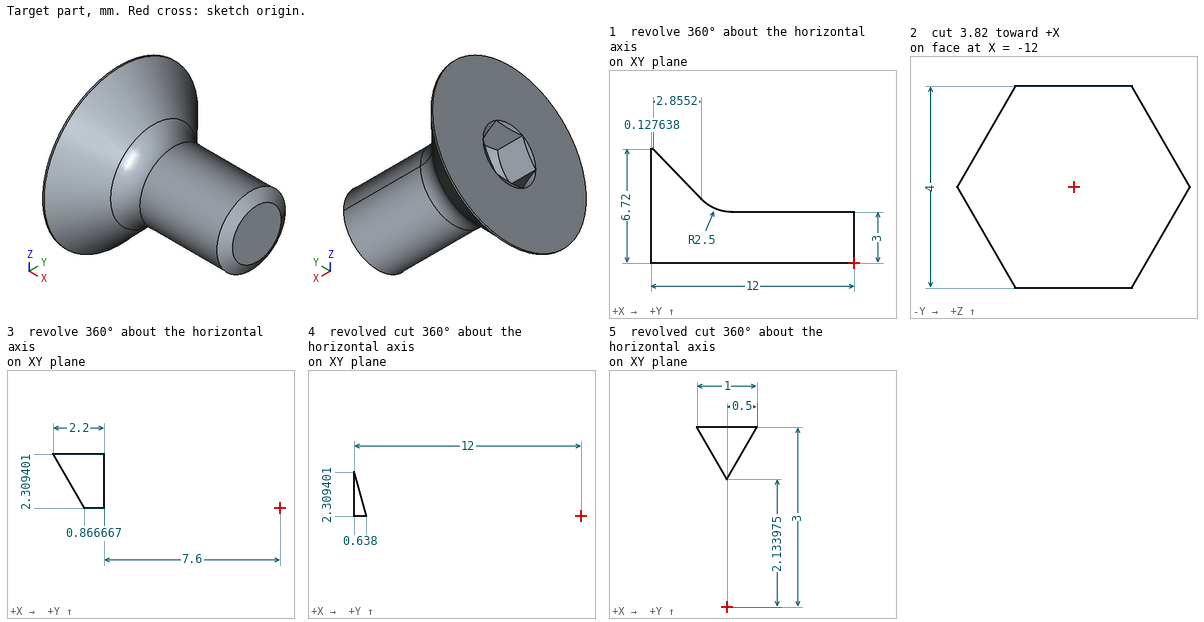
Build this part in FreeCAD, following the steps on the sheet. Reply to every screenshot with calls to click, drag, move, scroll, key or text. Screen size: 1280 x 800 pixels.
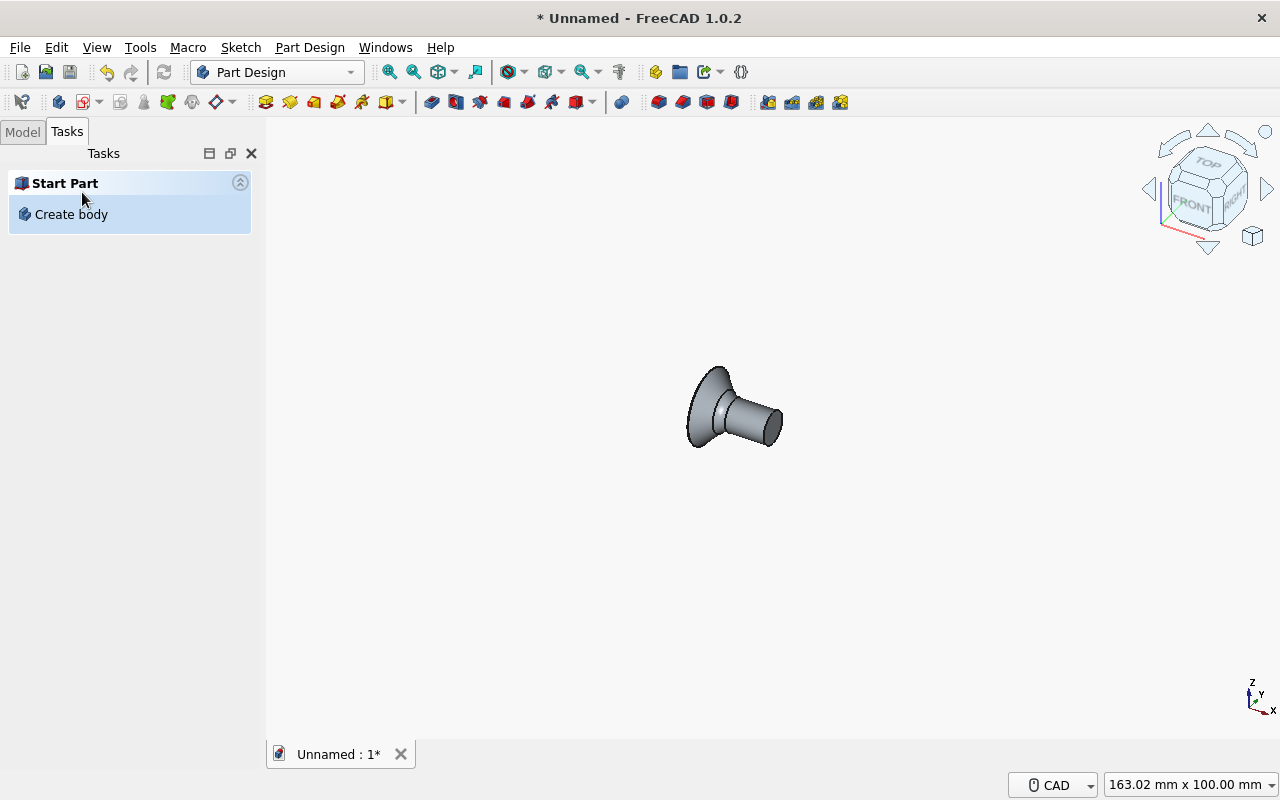
key(v)
key(f)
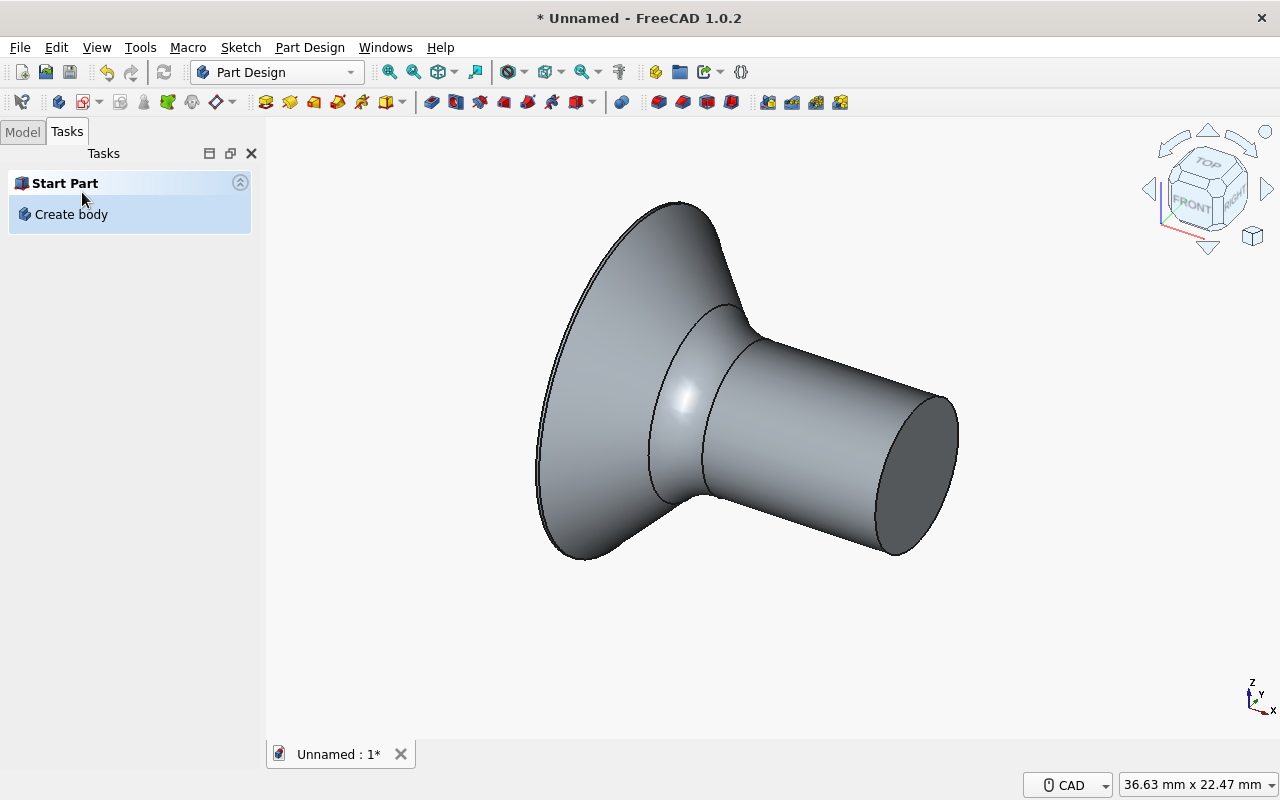
key(6)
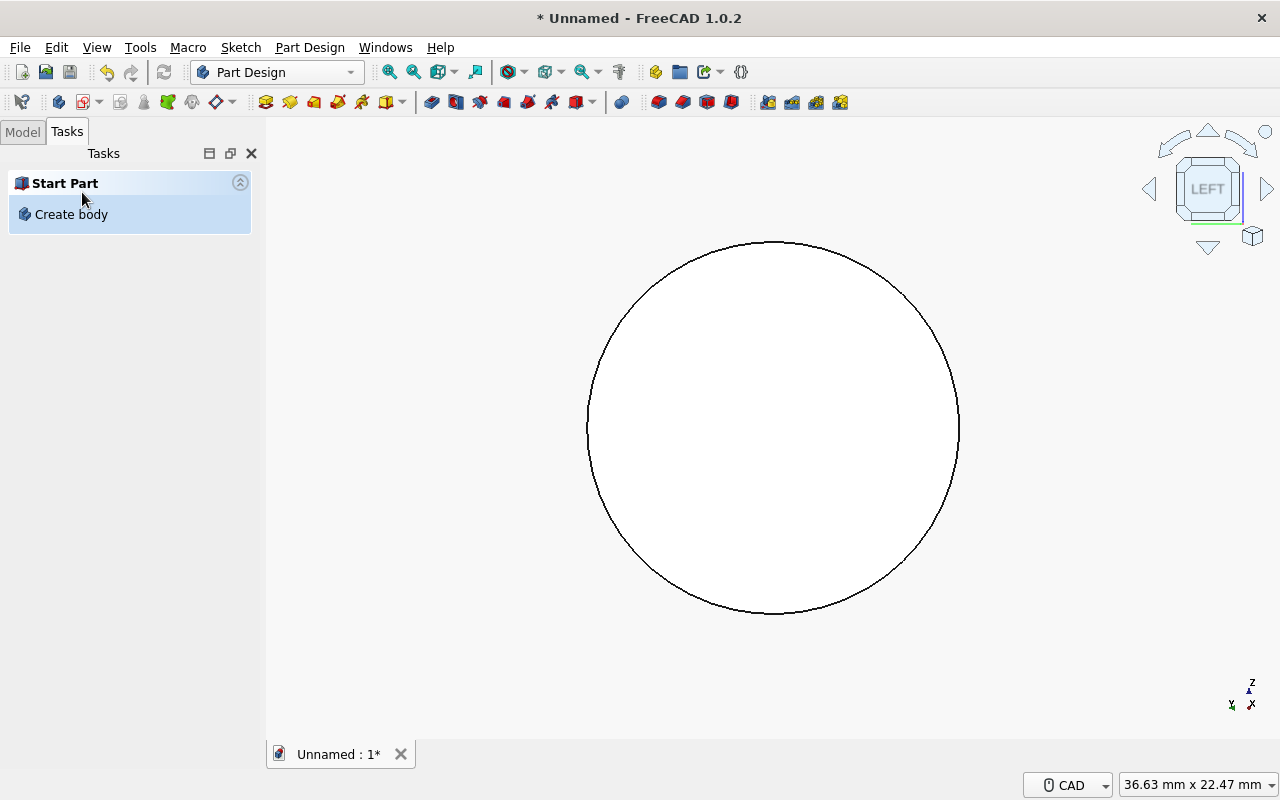
click(773, 427)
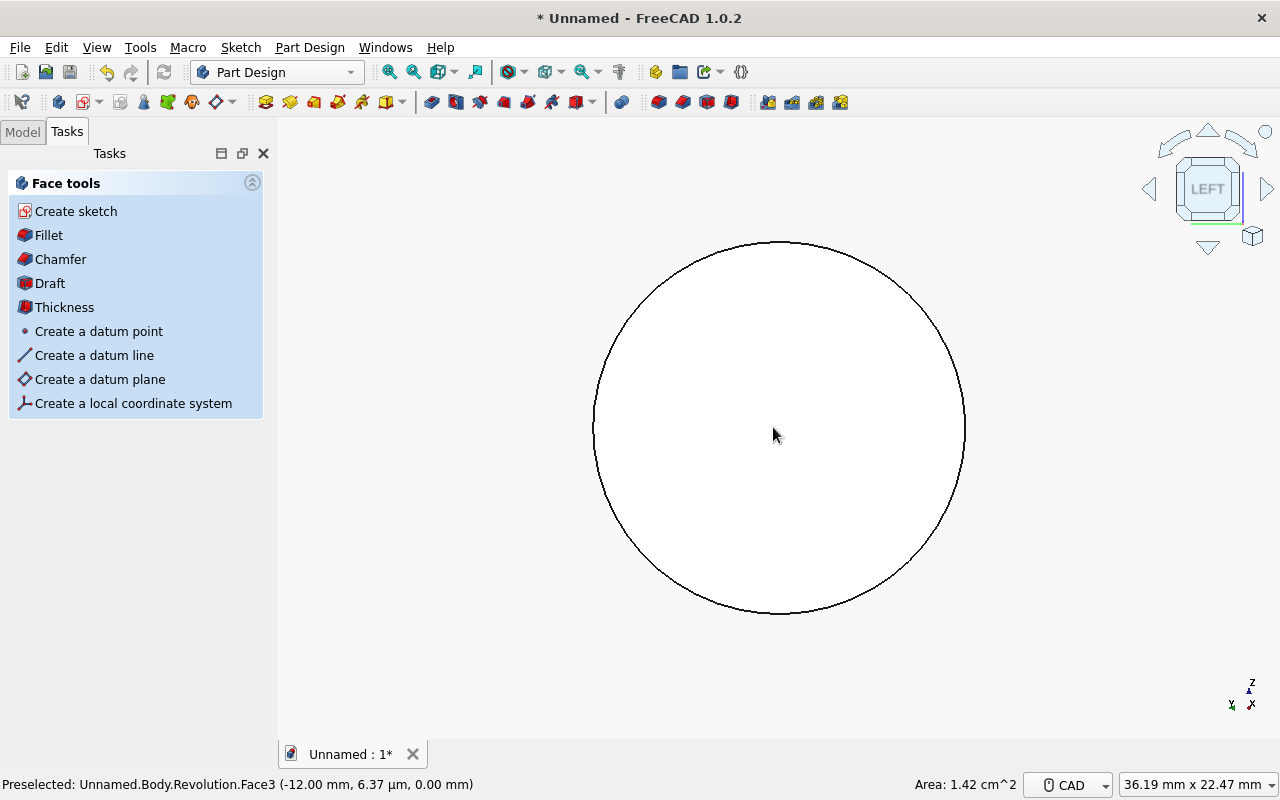
click(84, 102)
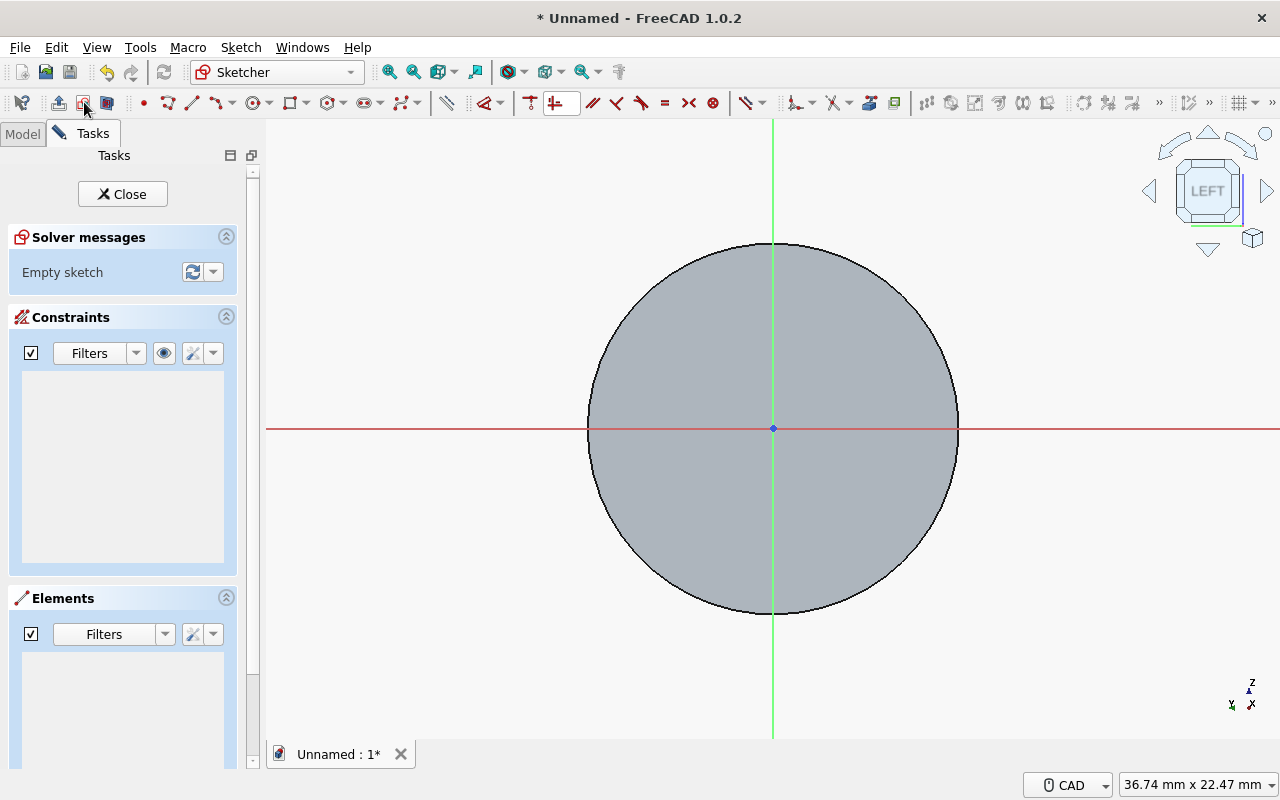
scroll(803, 429, up, 6)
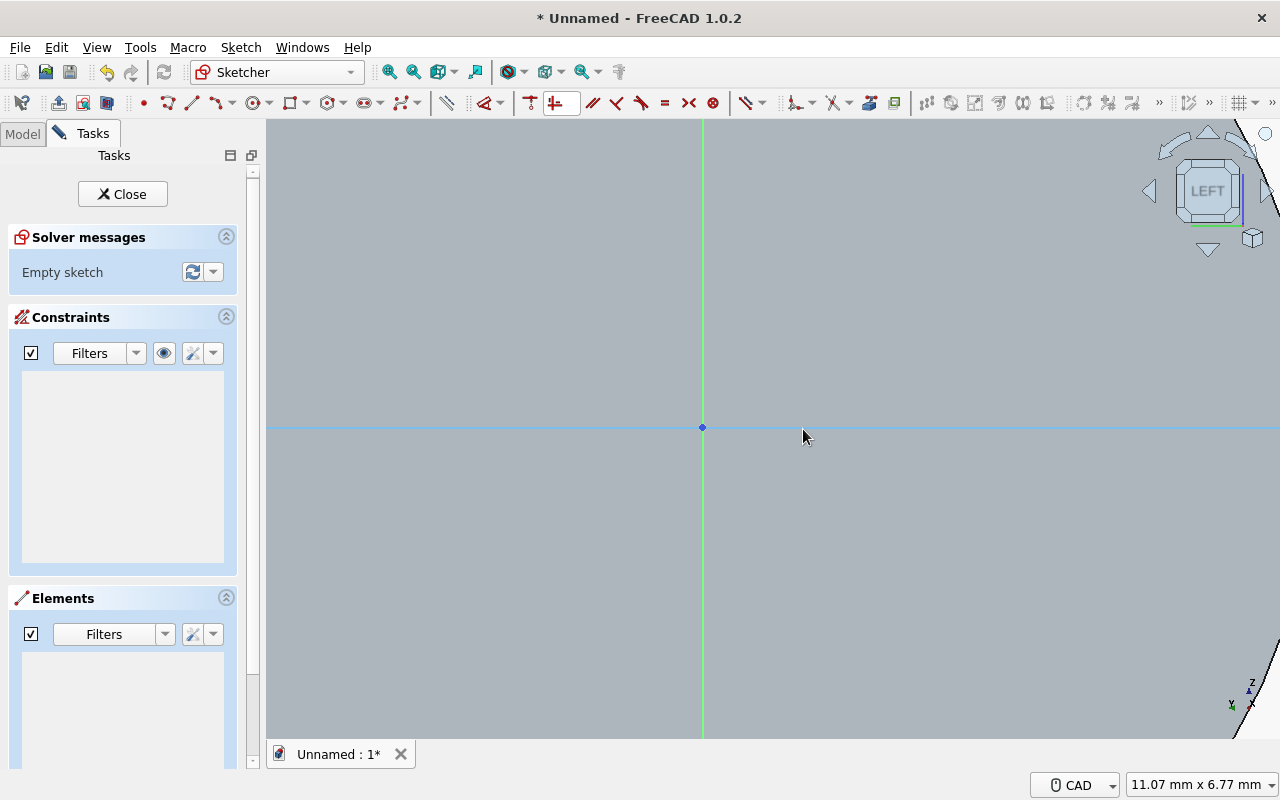
key(g)
key(p)
key(6)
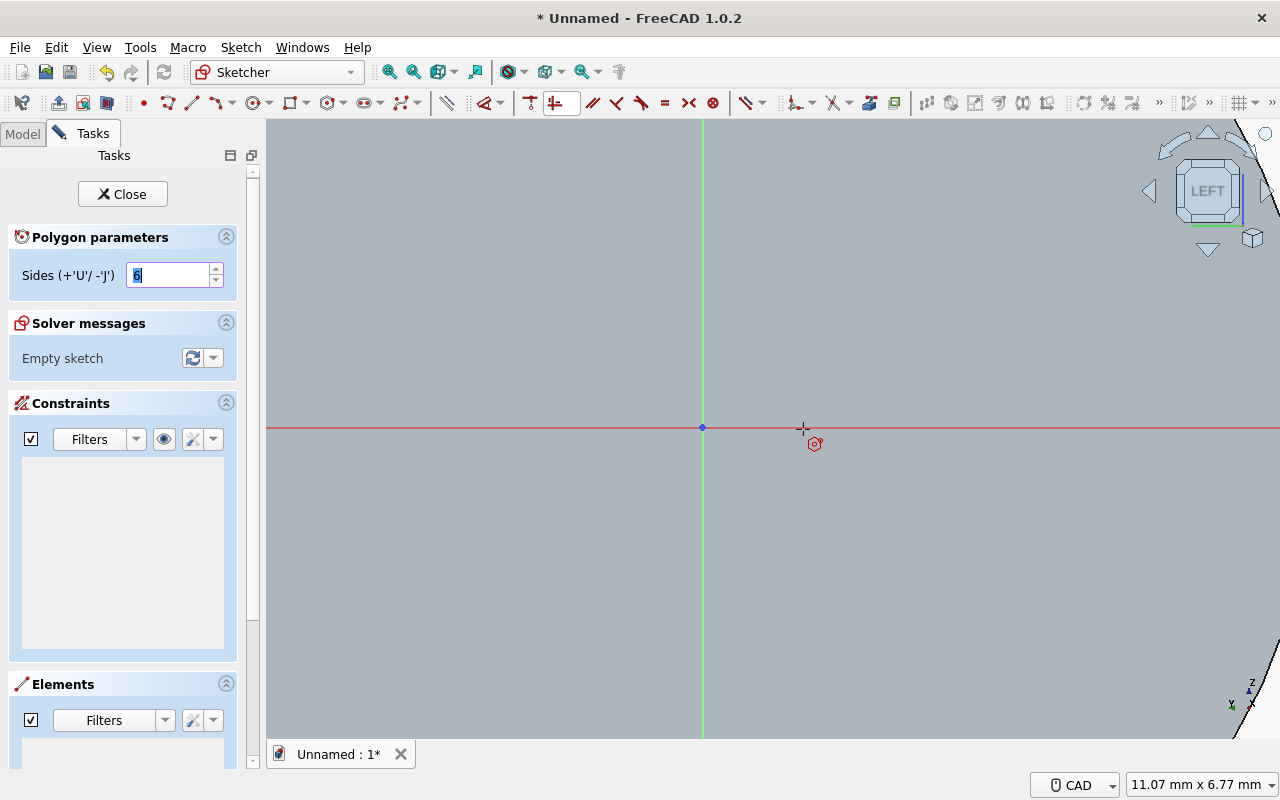
click(703, 428)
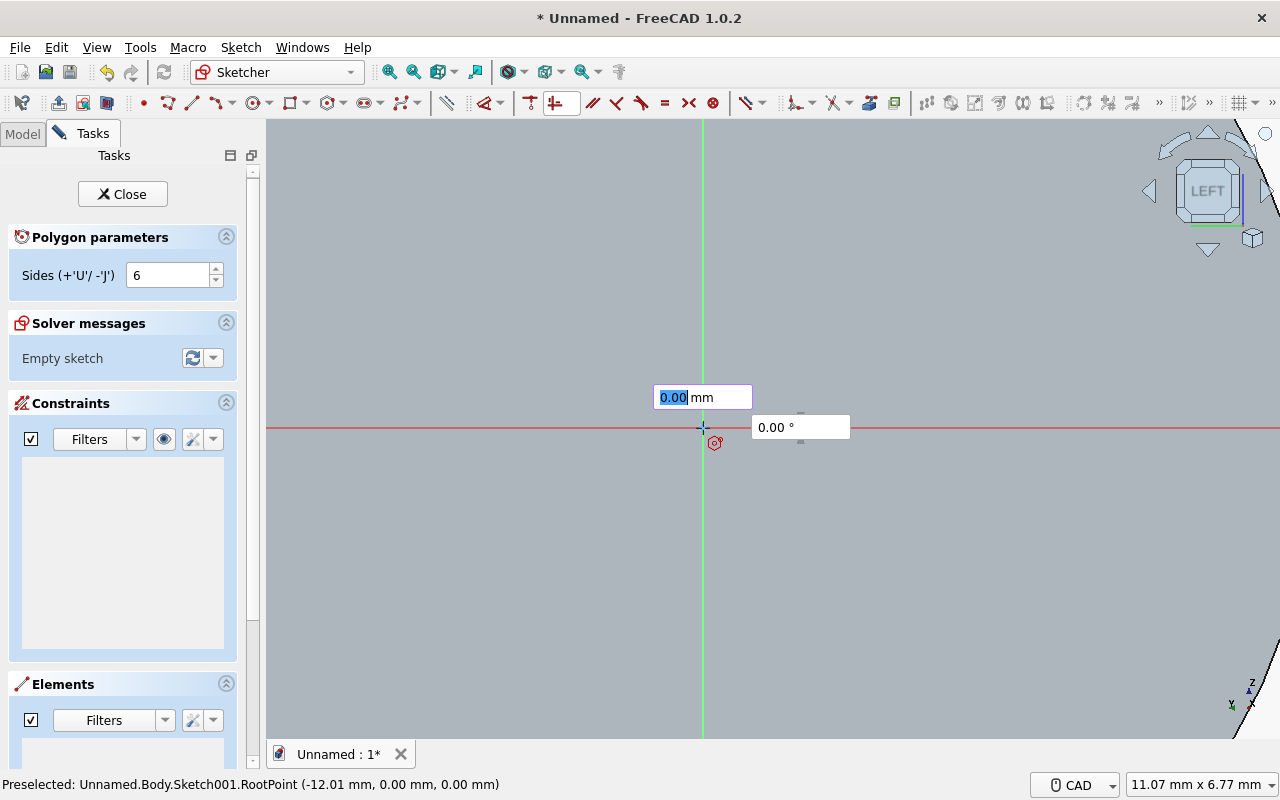
click(491, 428)
right_click(491, 428)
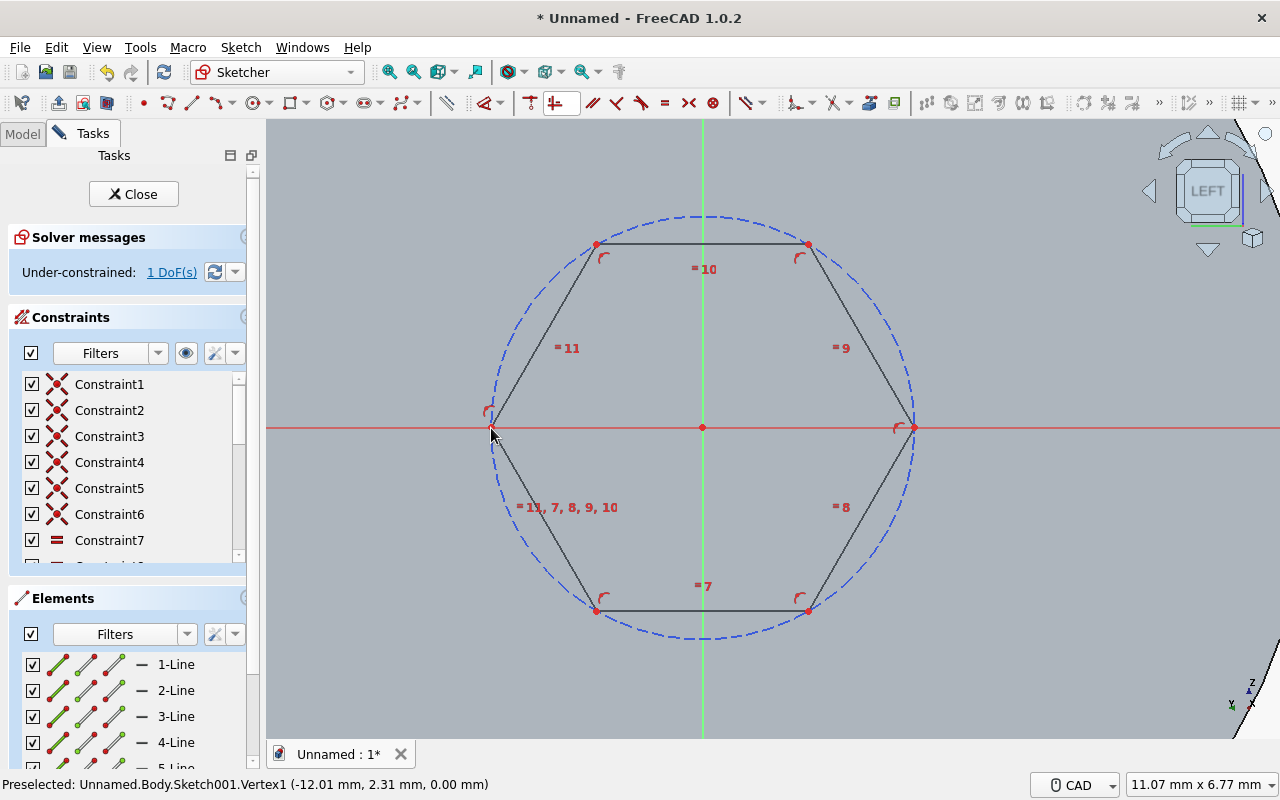
click(484, 104)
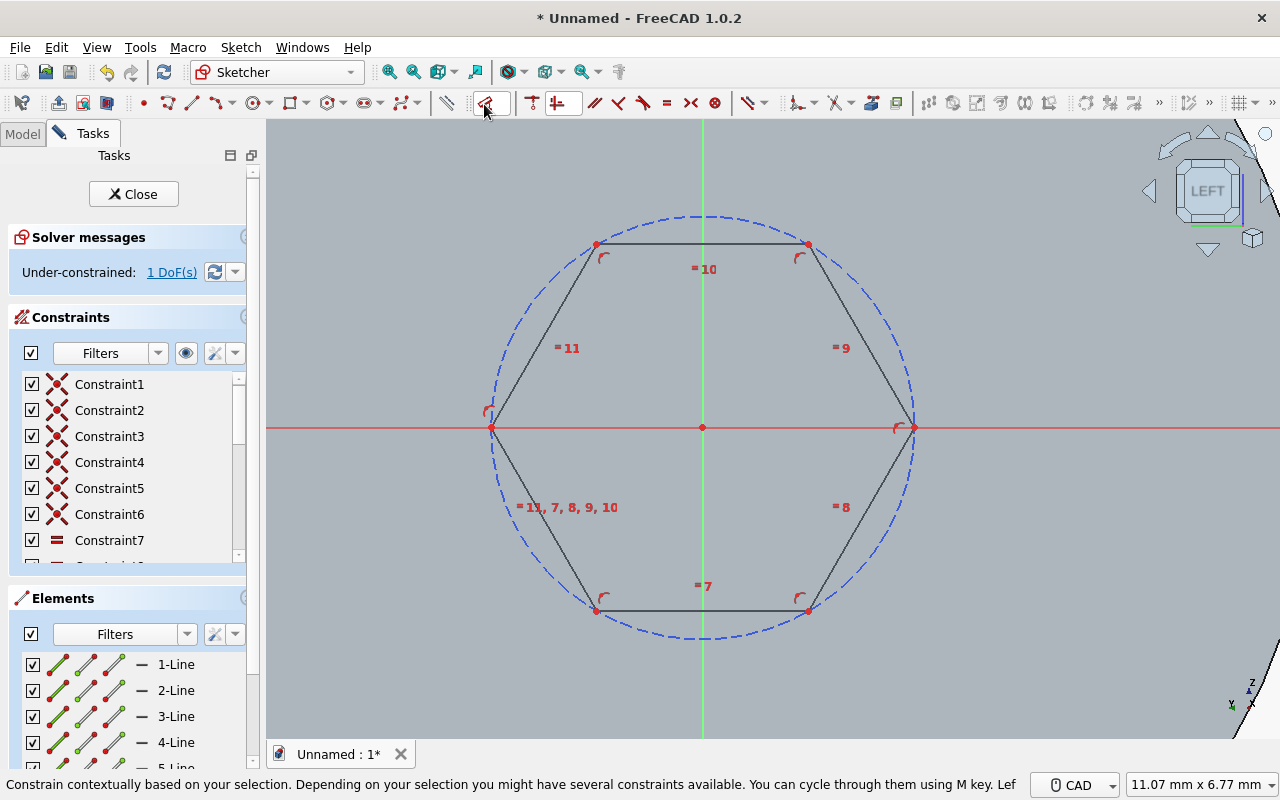
click(597, 611)